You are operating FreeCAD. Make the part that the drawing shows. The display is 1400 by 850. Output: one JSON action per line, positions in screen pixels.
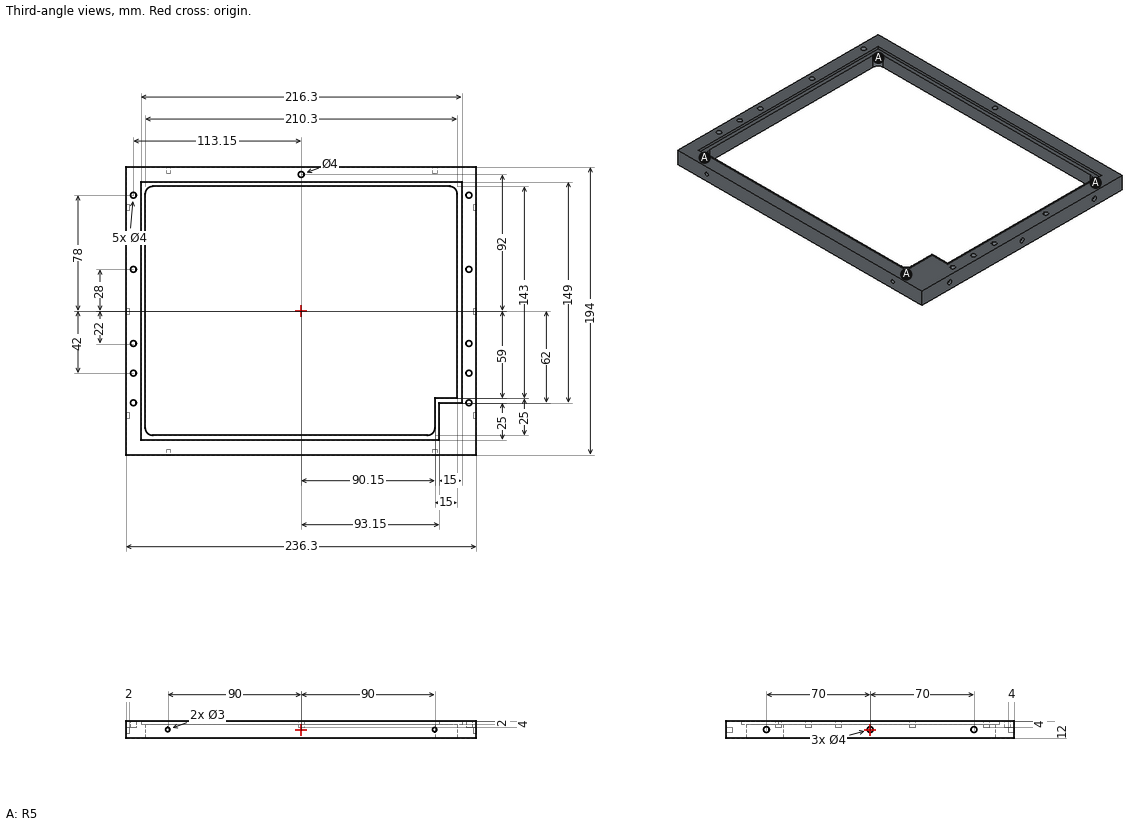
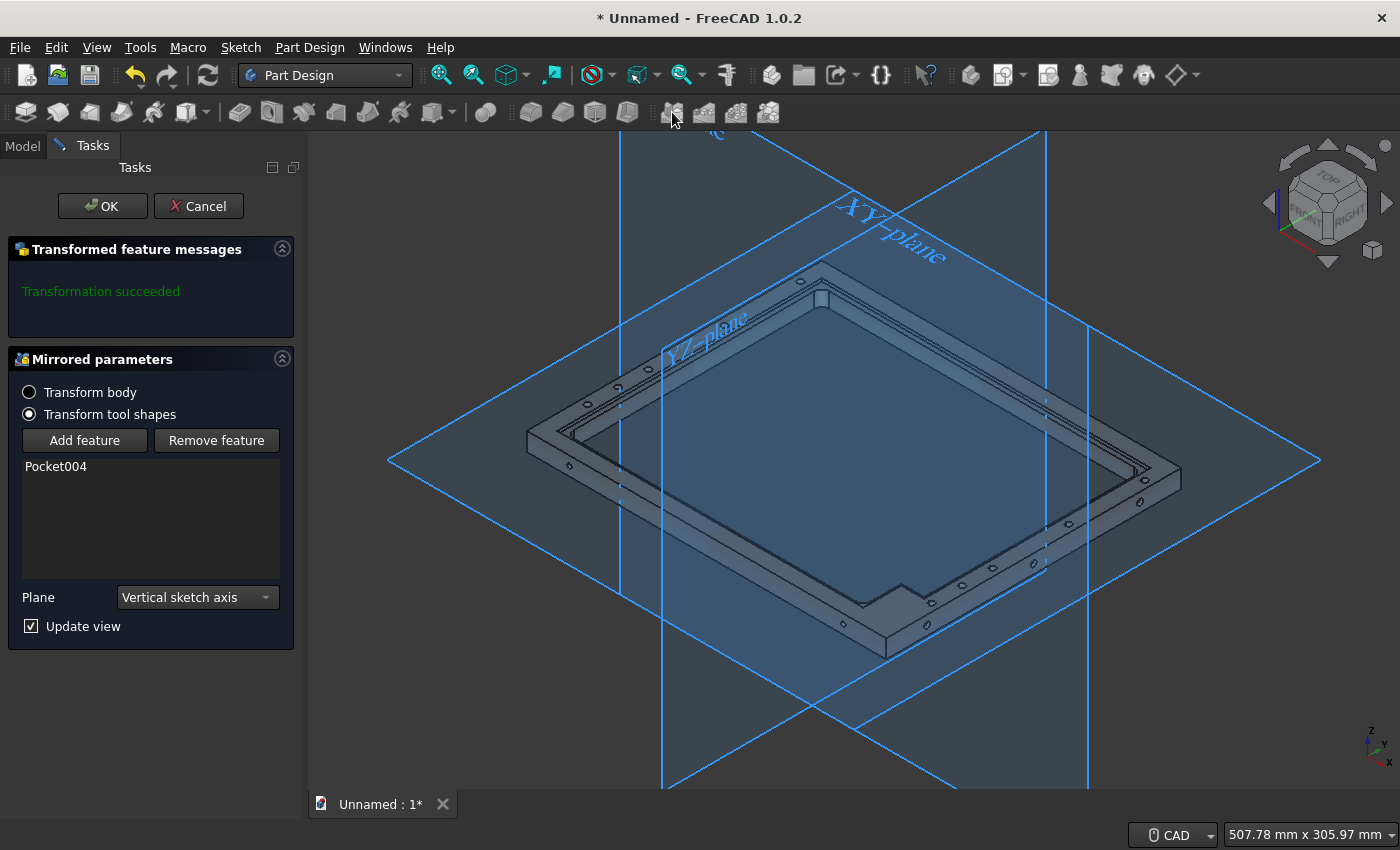
{"action": "left_click", "coordinate": [198, 598]}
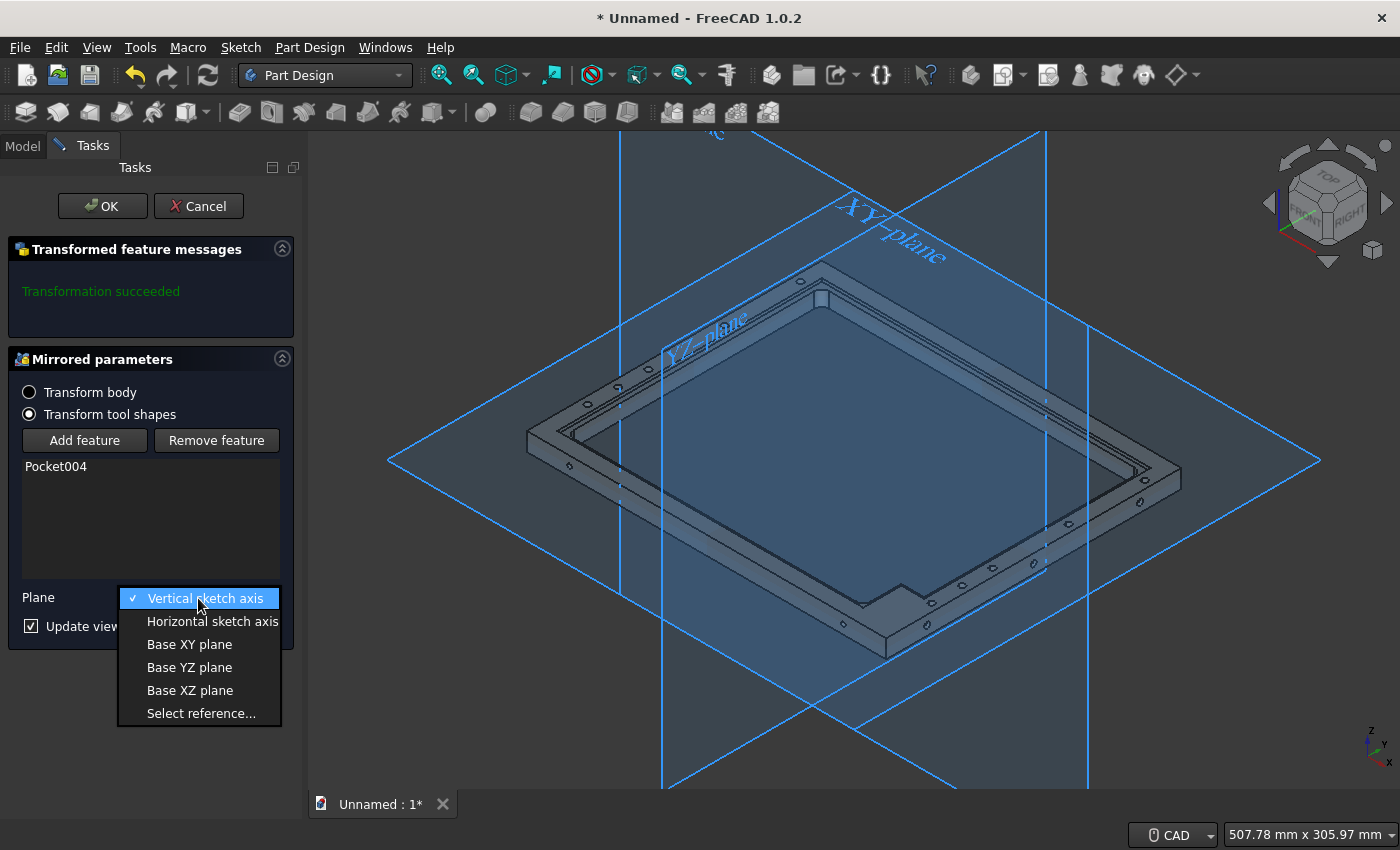
{"action": "left_click", "coordinate": [198, 668]}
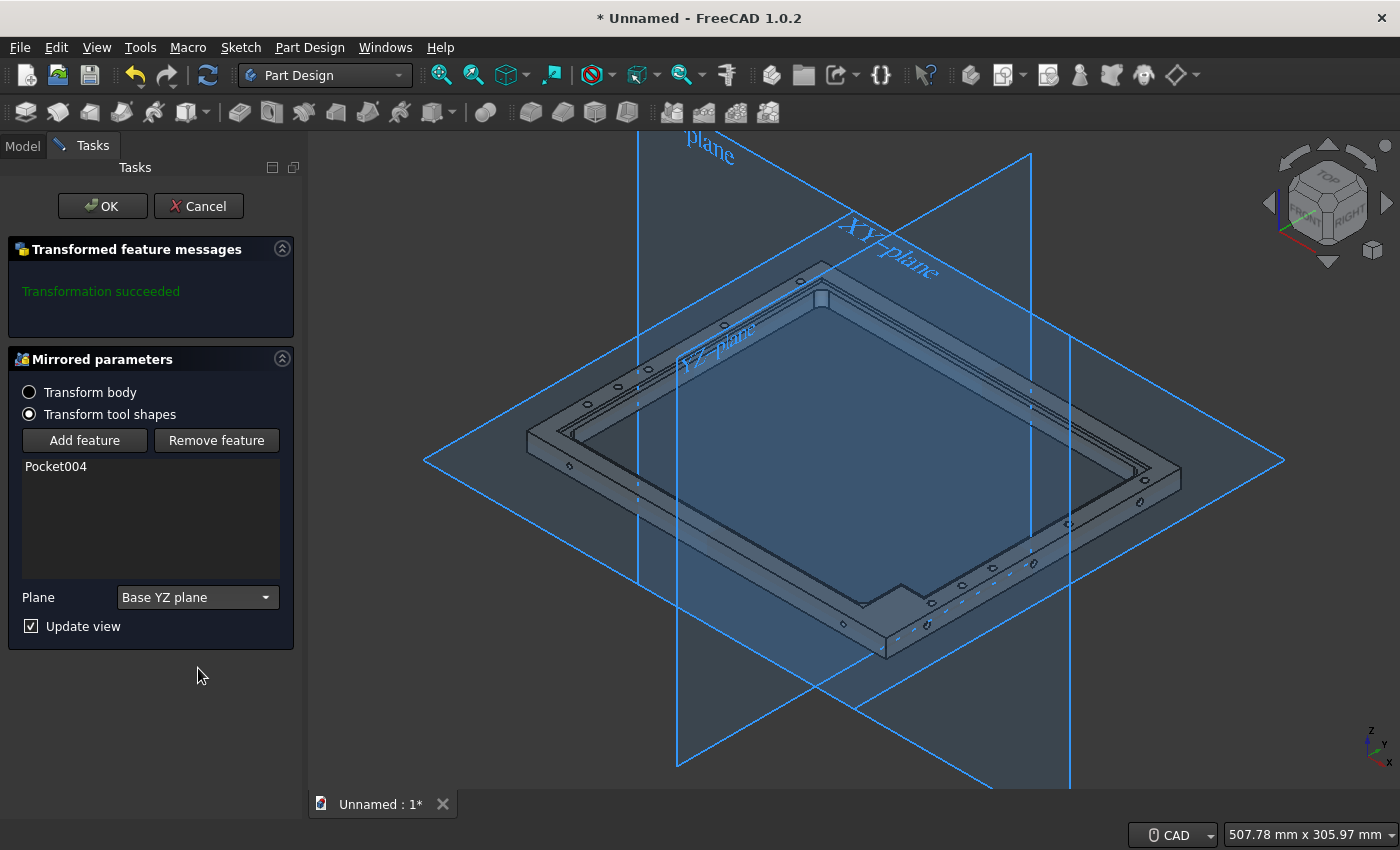
{"action": "left_click", "coordinate": [103, 206]}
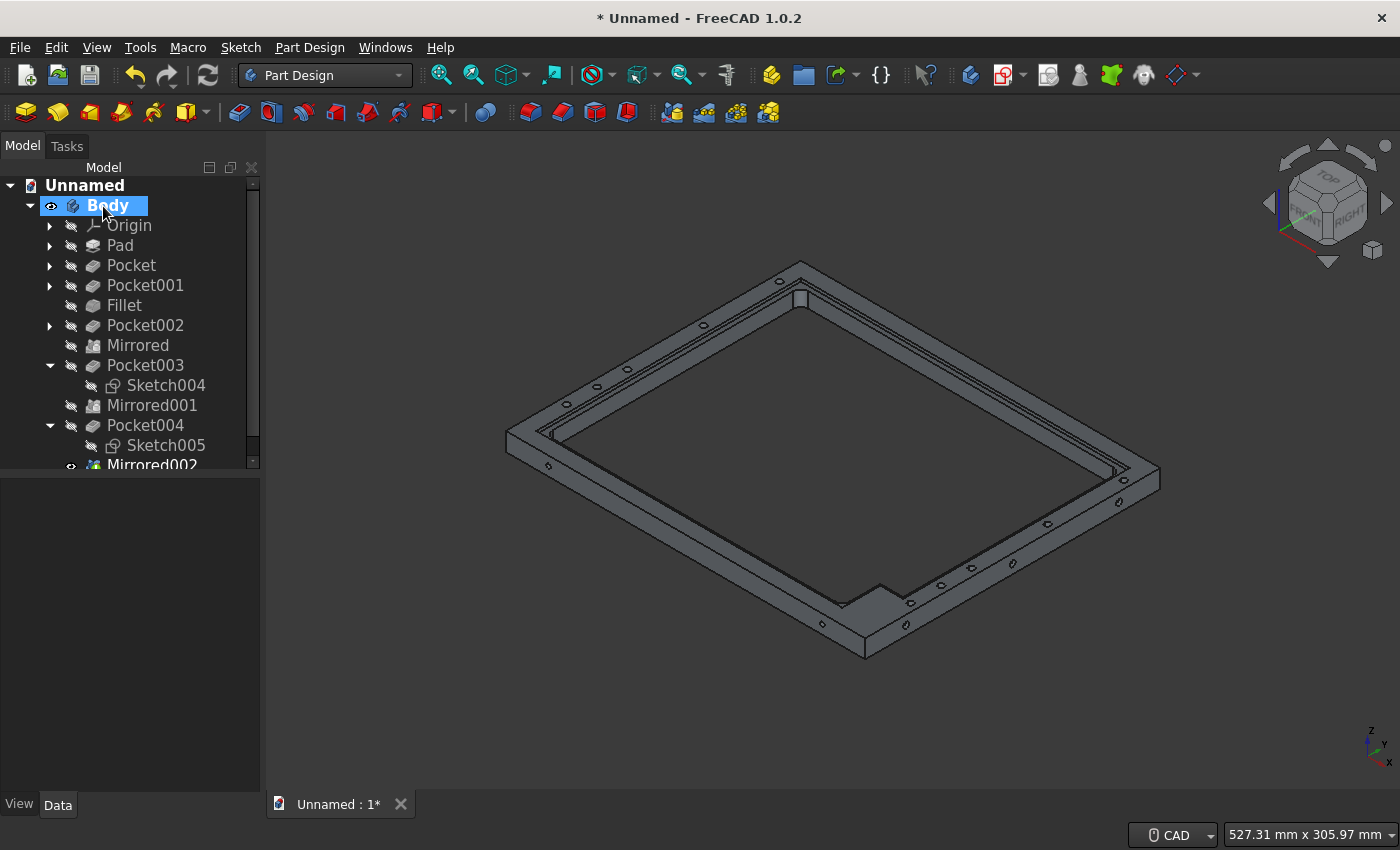
{"action": "left_click", "coordinate": [861, 610]}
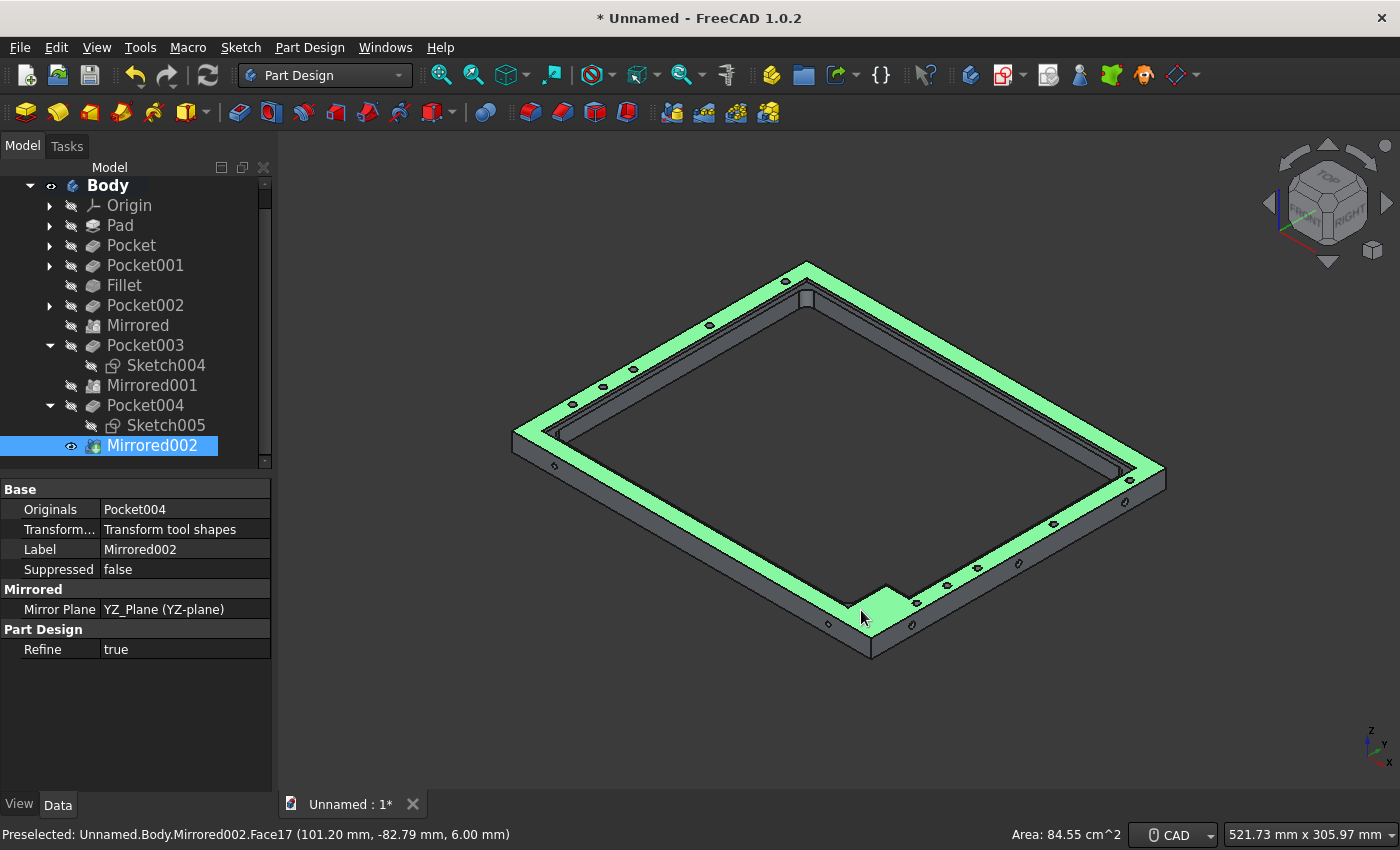
{"action": "left_click", "coordinate": [1004, 76]}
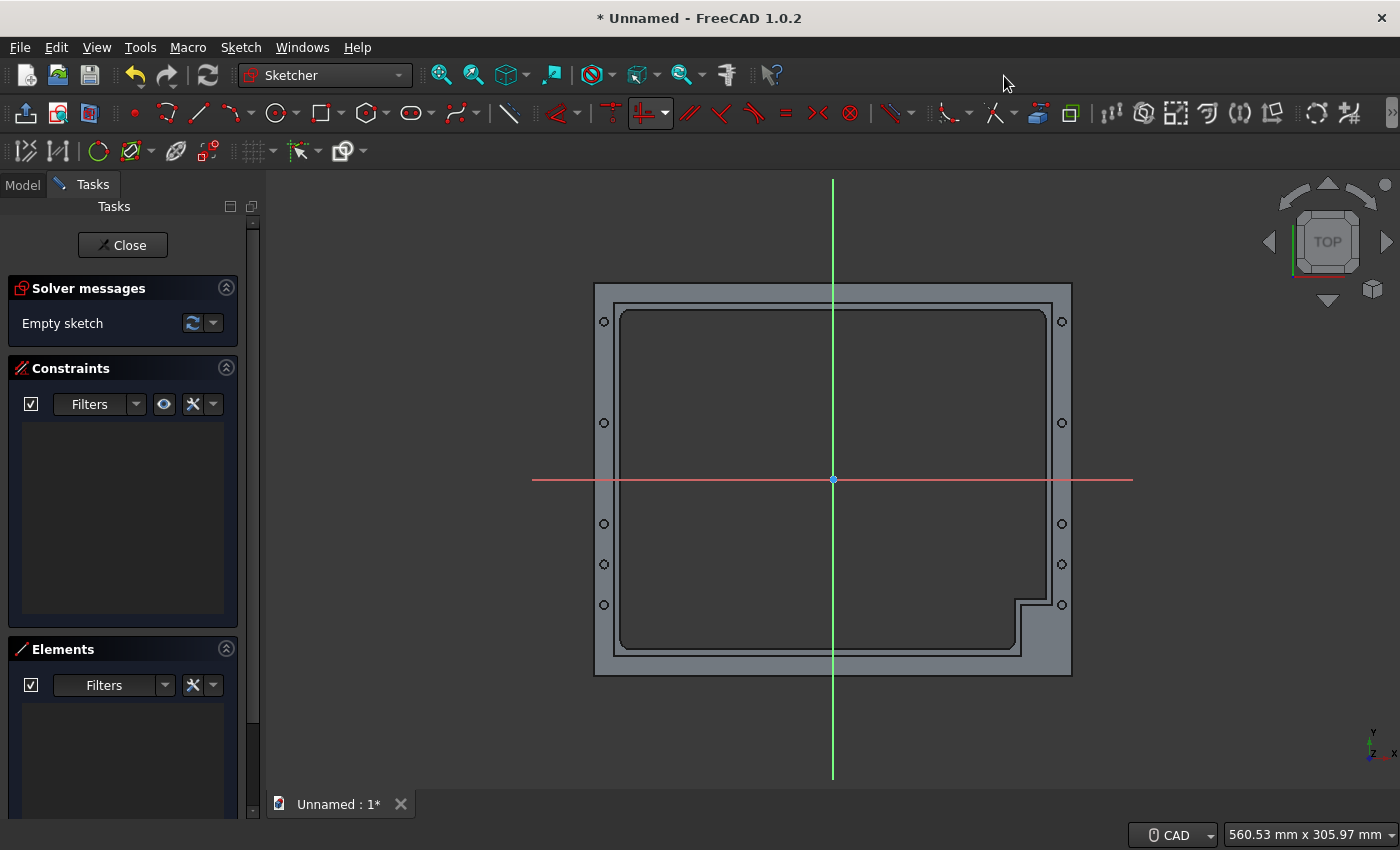
{"action": "scroll", "coordinate": [837, 284], "scroll_direction": "up", "scroll_amount": 15}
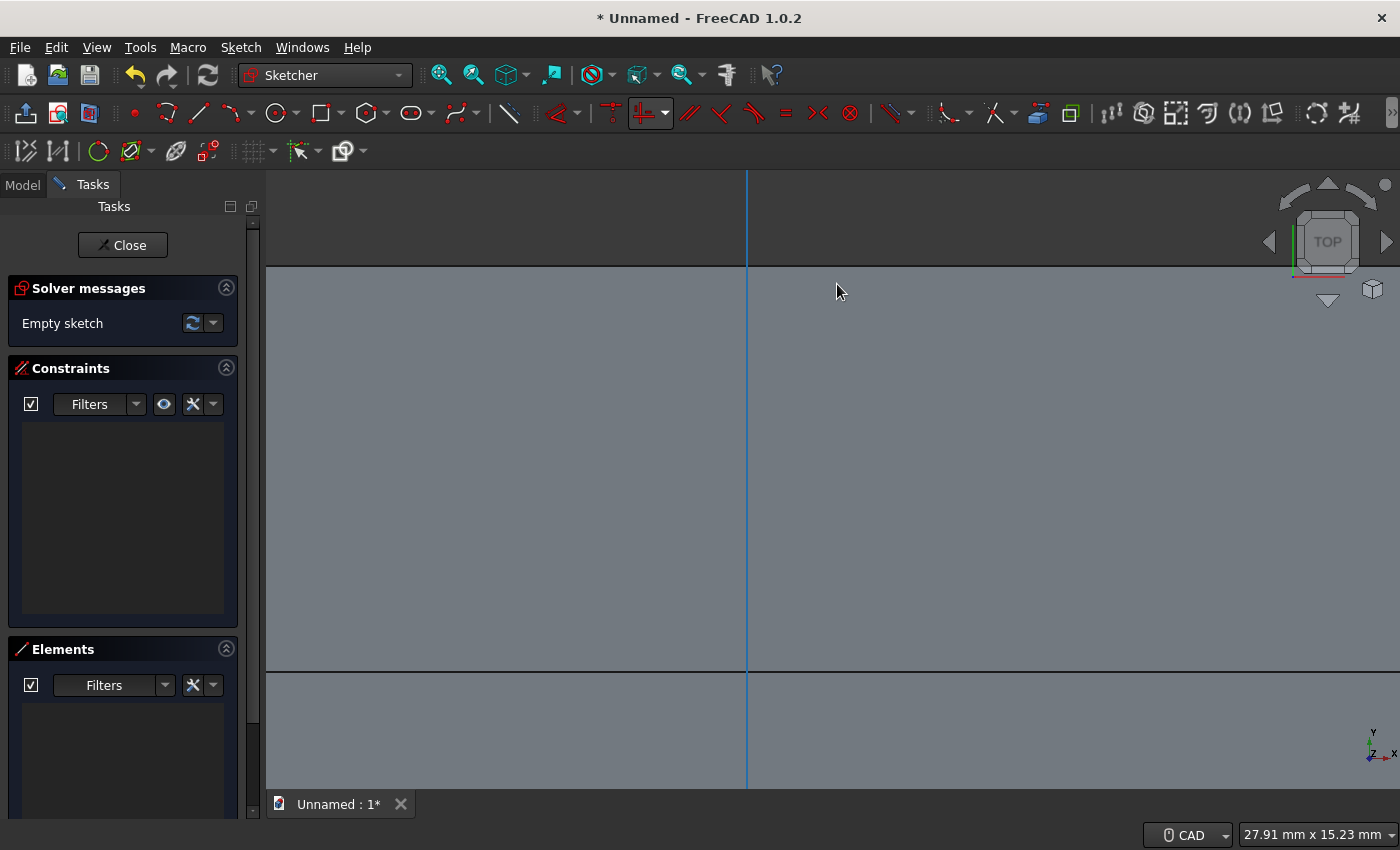
{"action": "scroll", "coordinate": [733, 460], "scroll_direction": "up", "scroll_amount": 4}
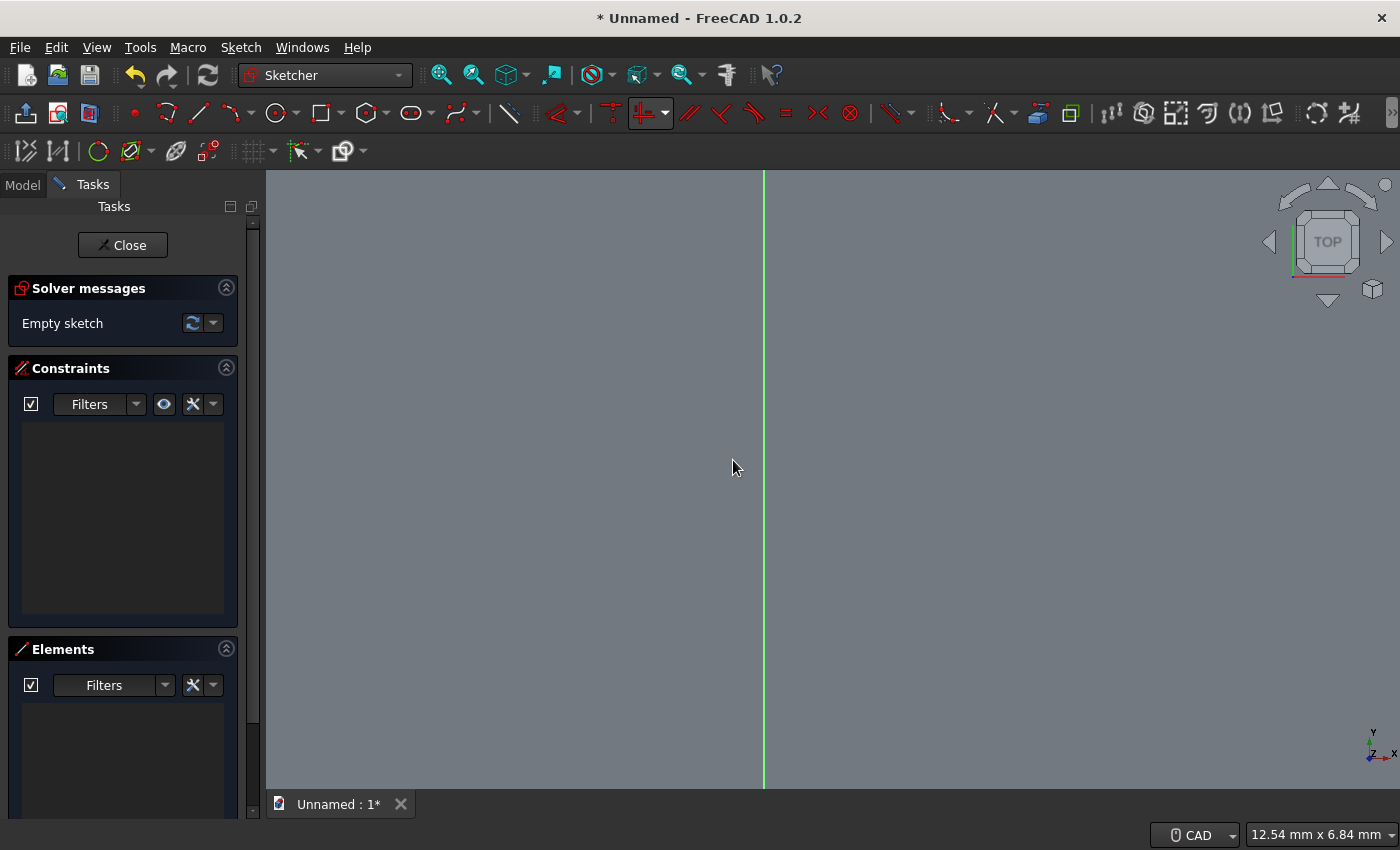
{"action": "left_click", "coordinate": [276, 114]}